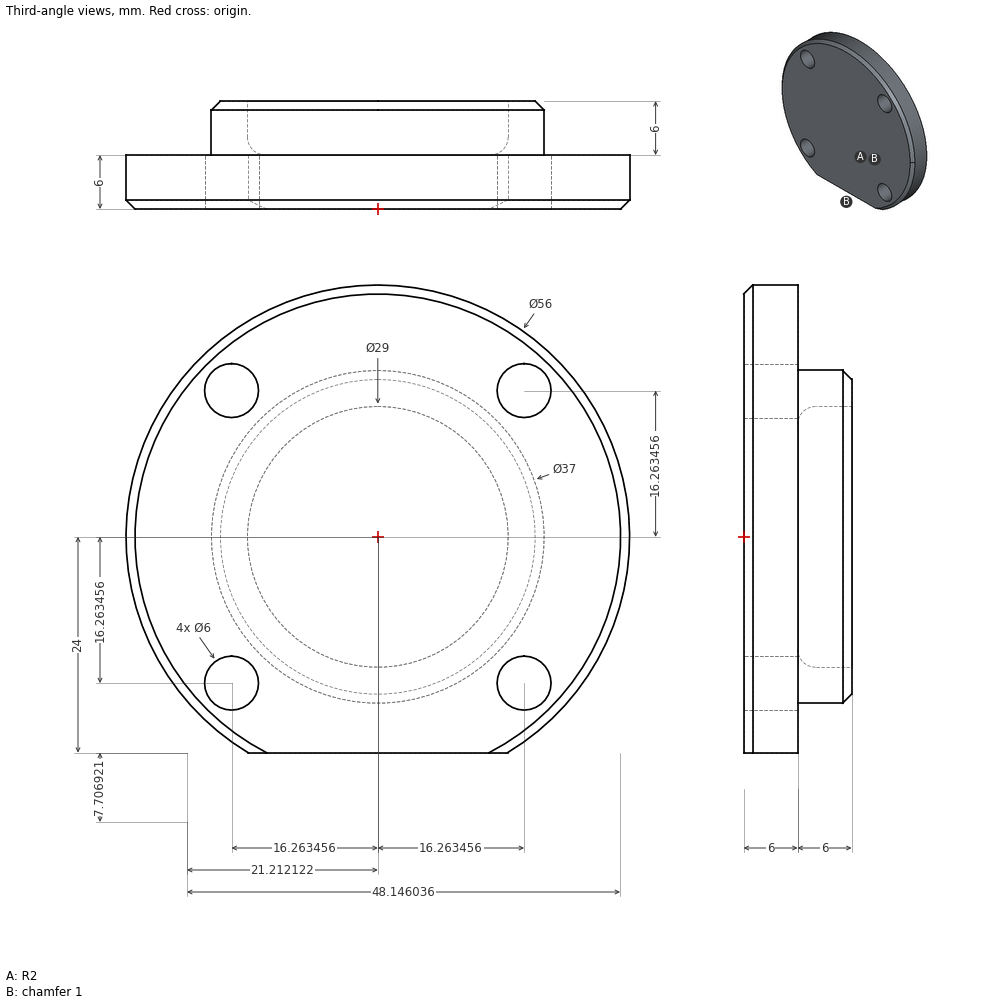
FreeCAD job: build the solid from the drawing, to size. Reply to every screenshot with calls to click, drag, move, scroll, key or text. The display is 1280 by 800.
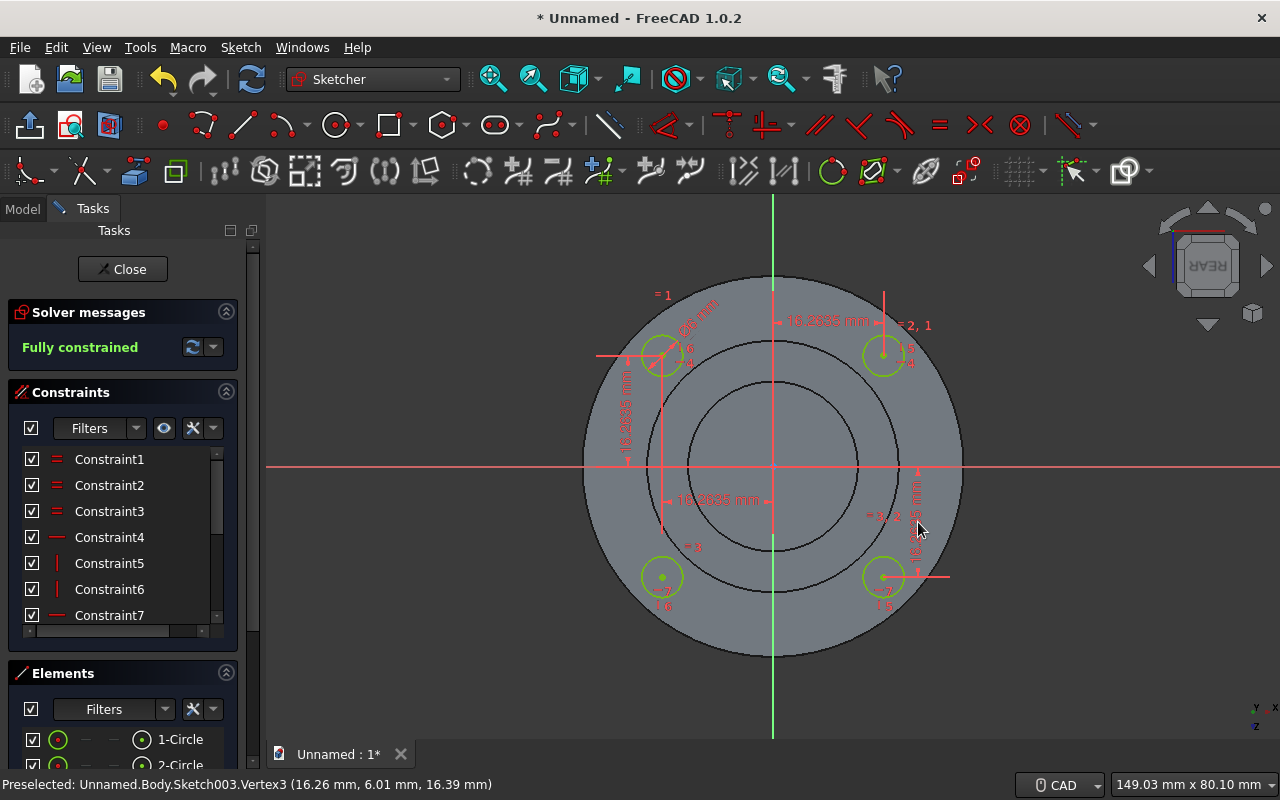
click(123, 269)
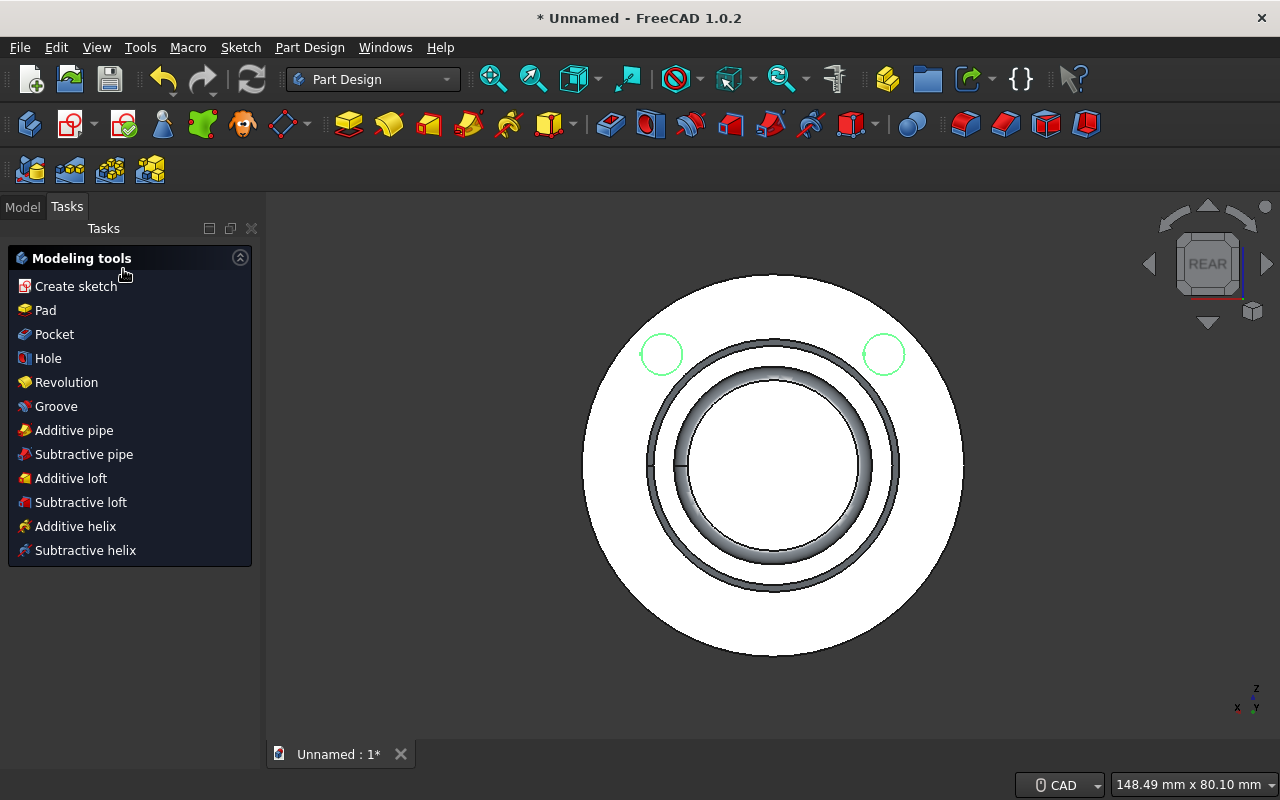
click(612, 124)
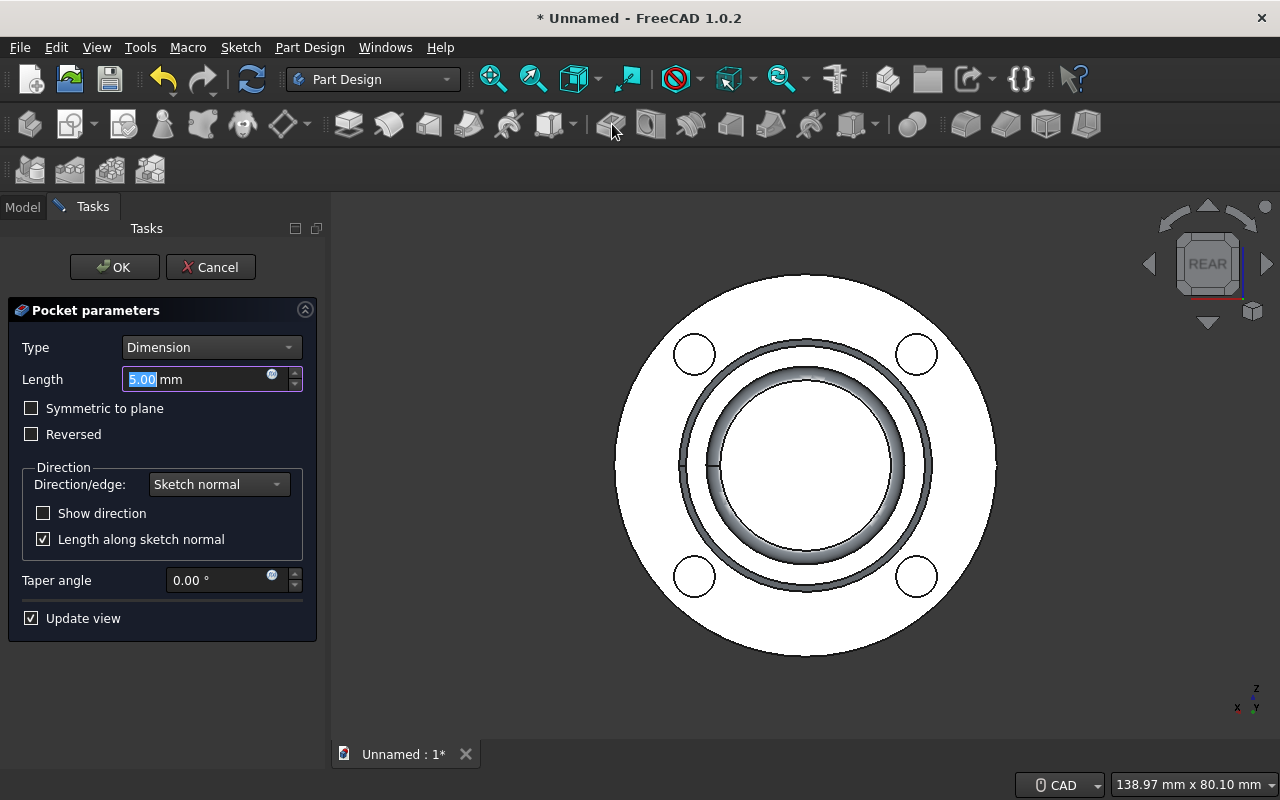
text(6)
key(Tab)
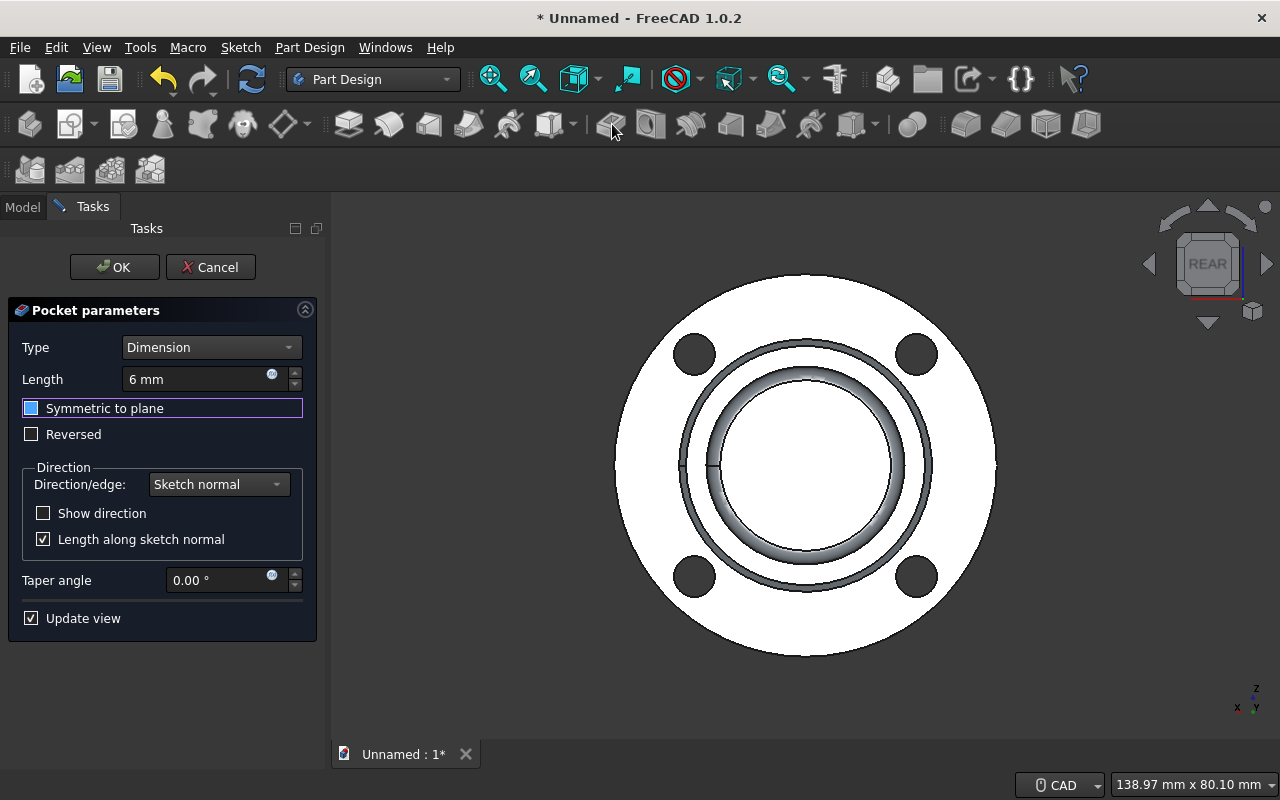
click(115, 267)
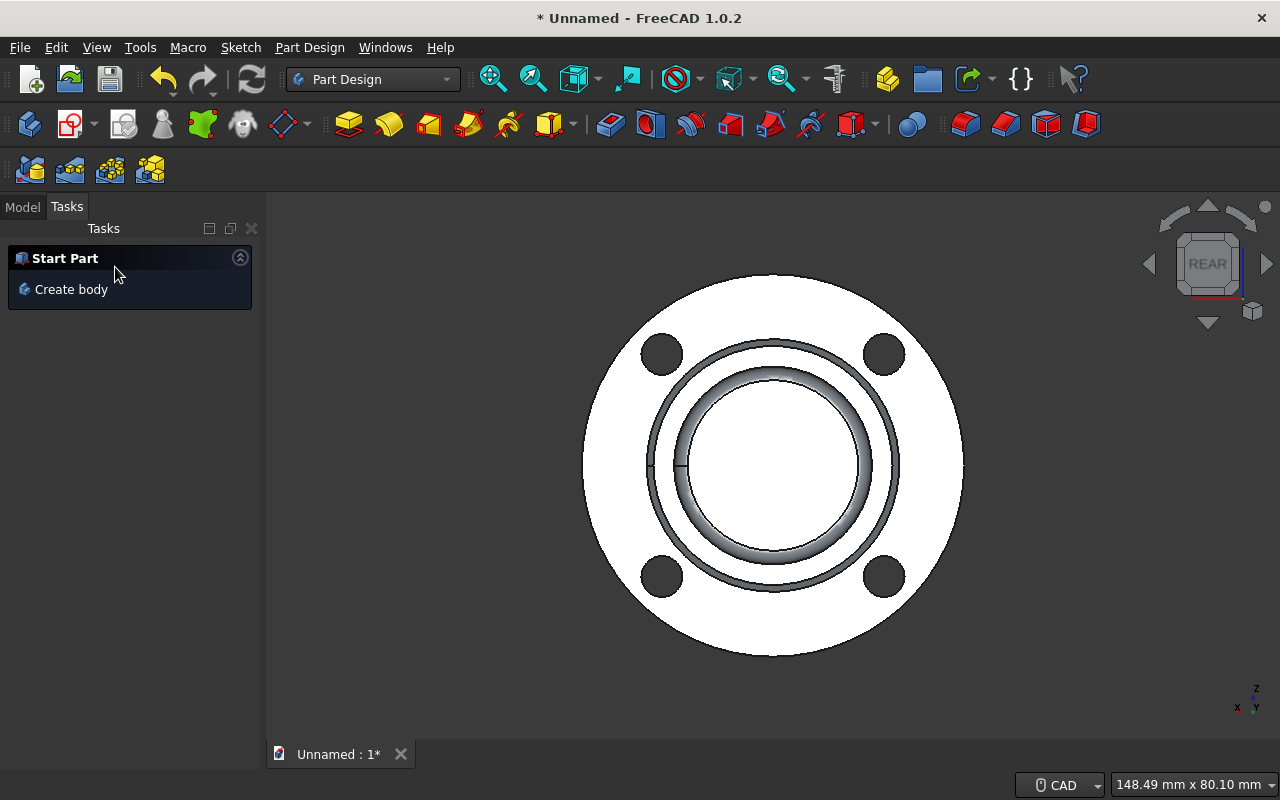
click(609, 464)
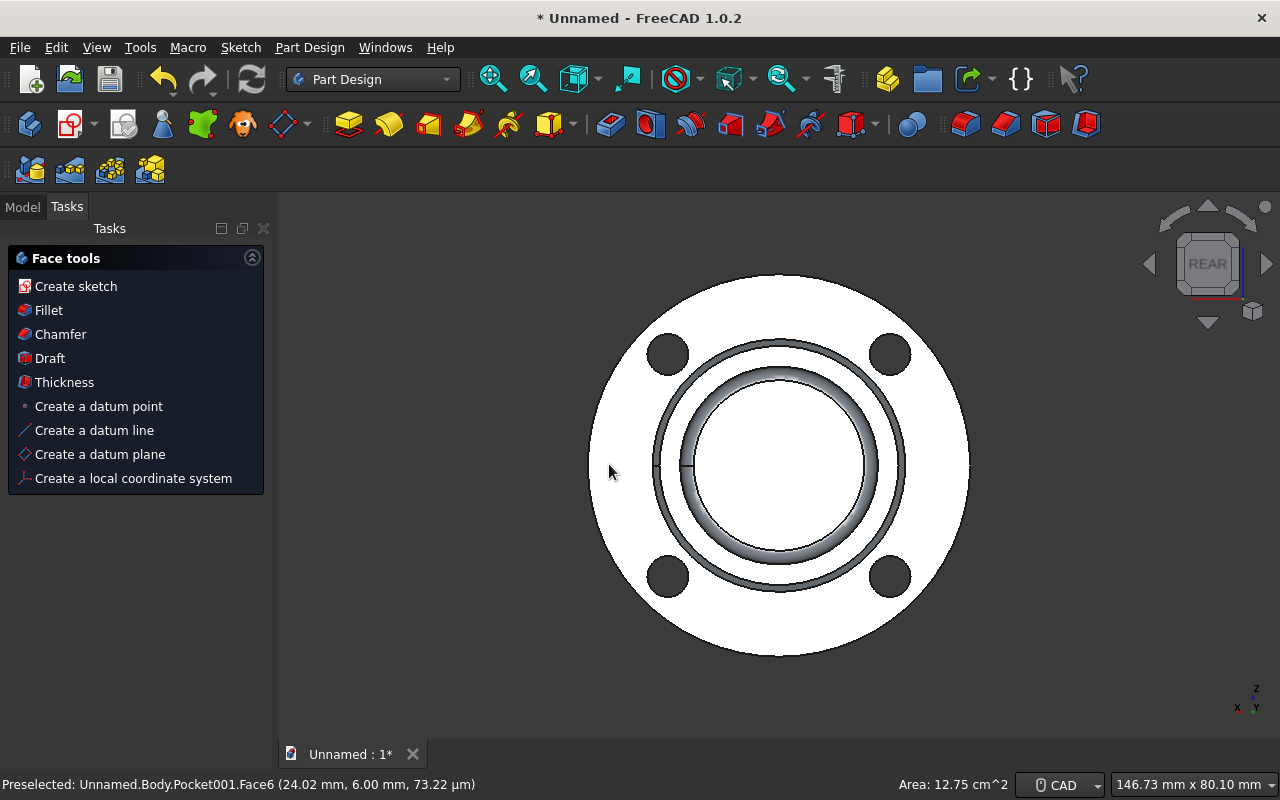
click(70, 124)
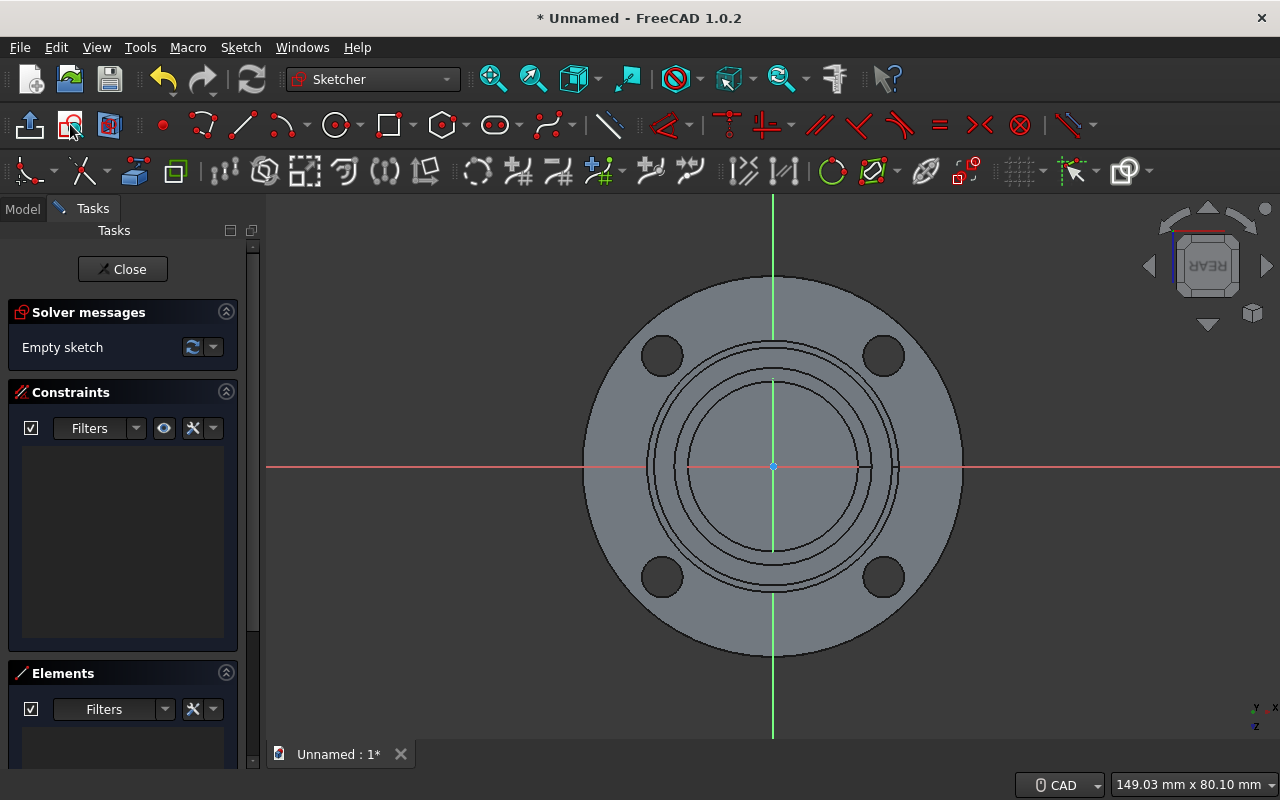
scroll(971, 222, up, 2)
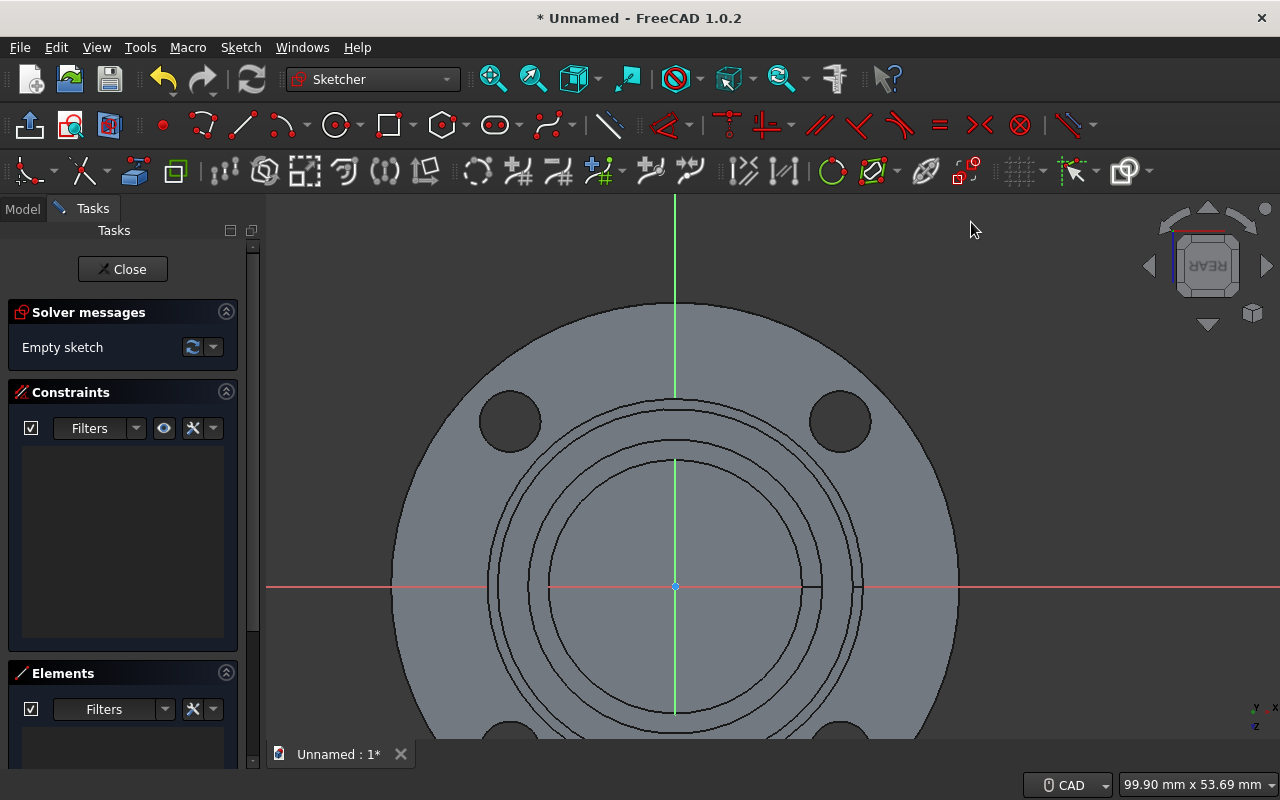
key(g)
key(r)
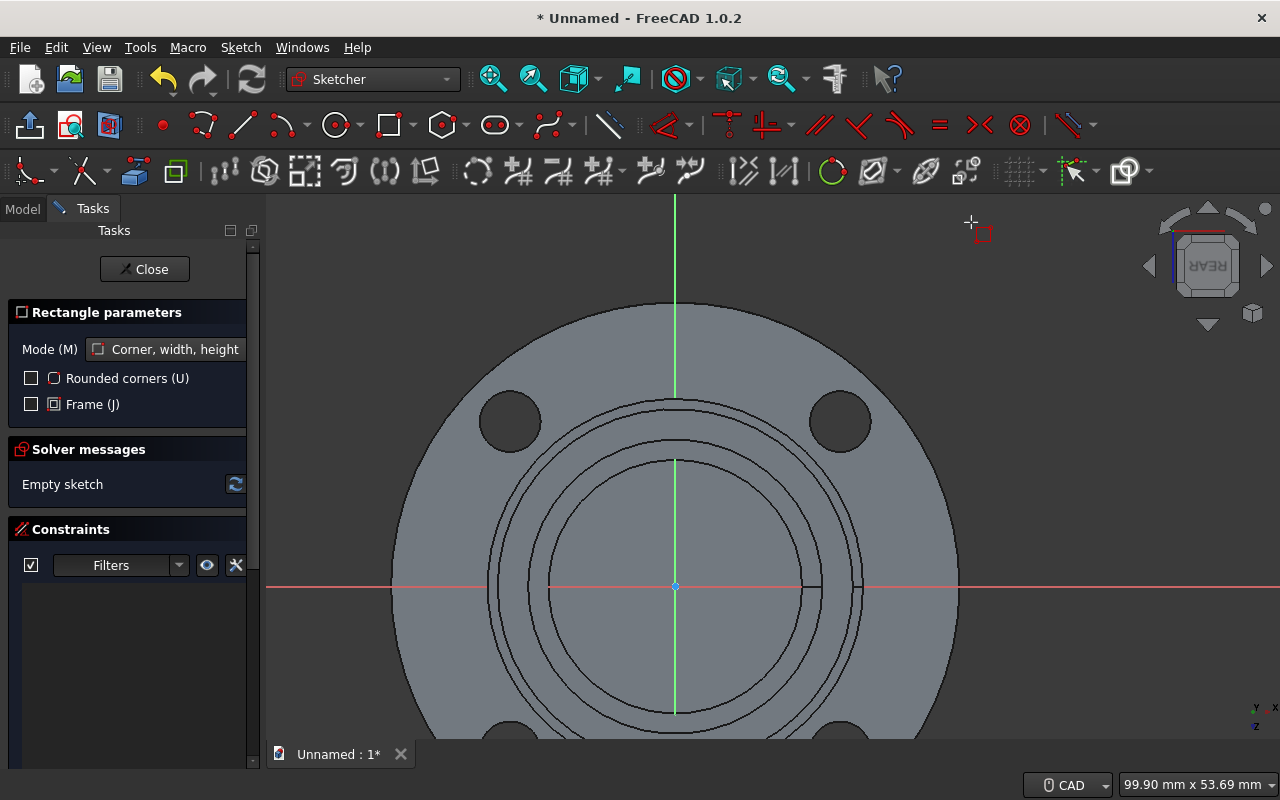
click(460, 265)
click(949, 343)
key(Escape)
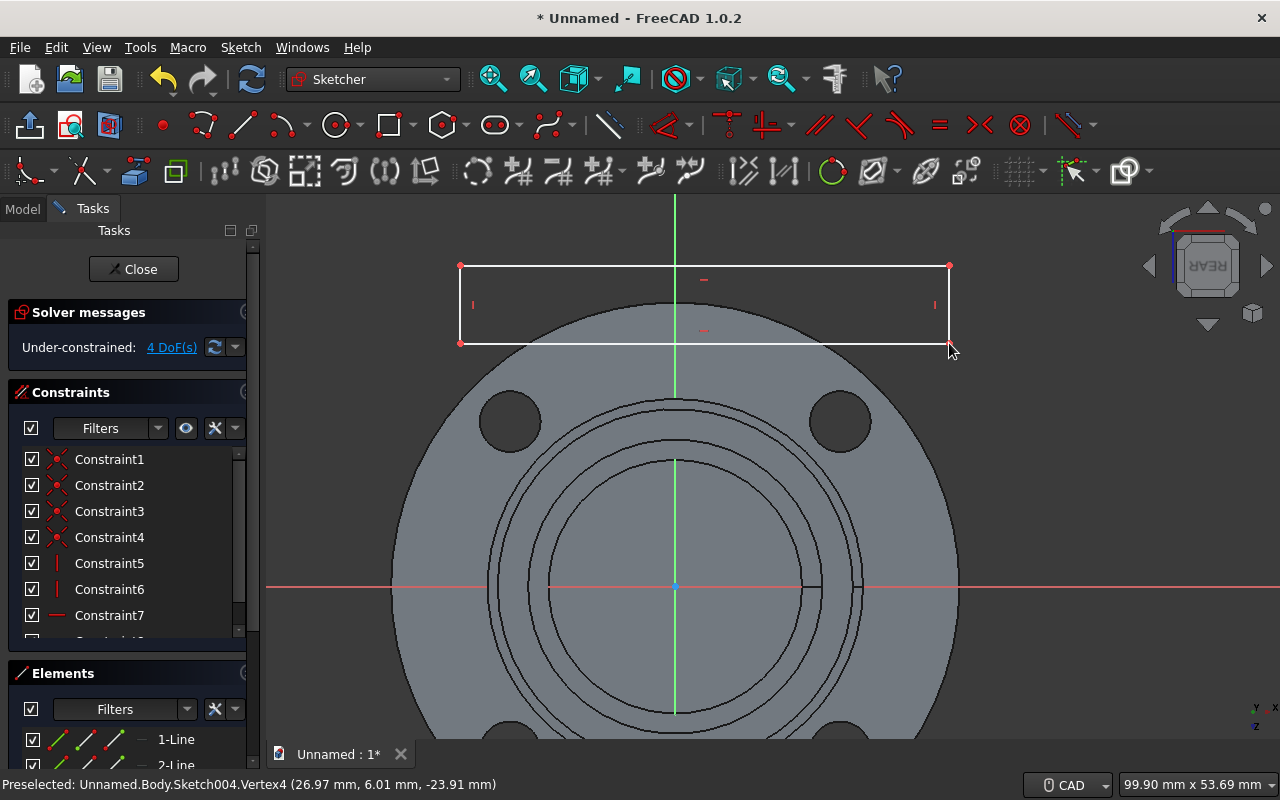
click(664, 126)